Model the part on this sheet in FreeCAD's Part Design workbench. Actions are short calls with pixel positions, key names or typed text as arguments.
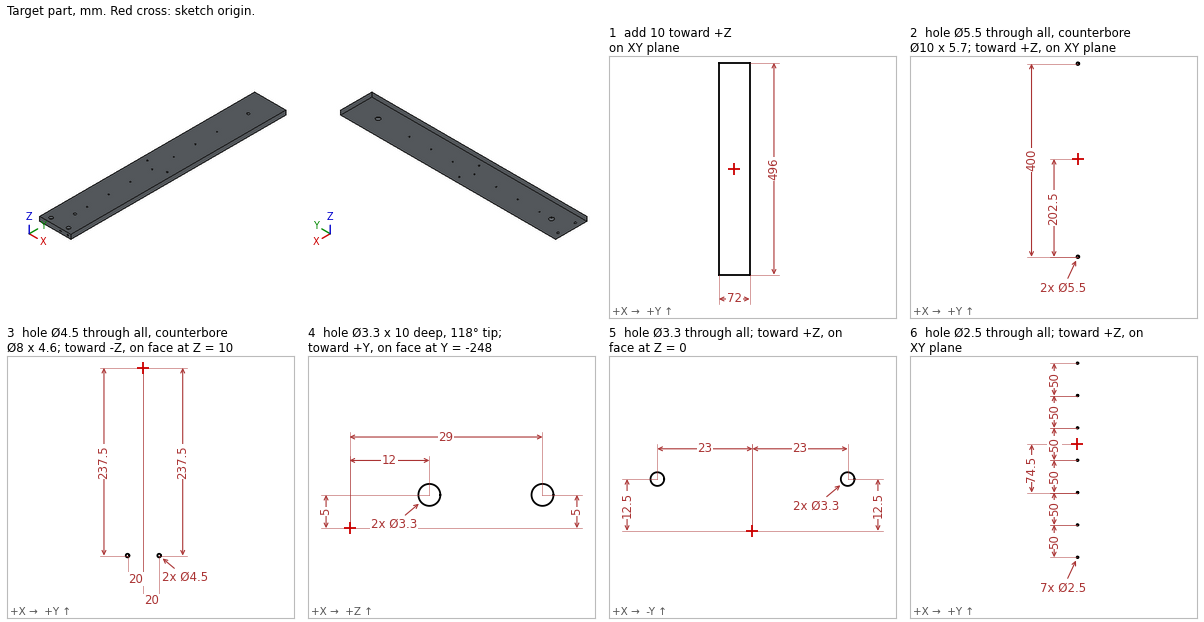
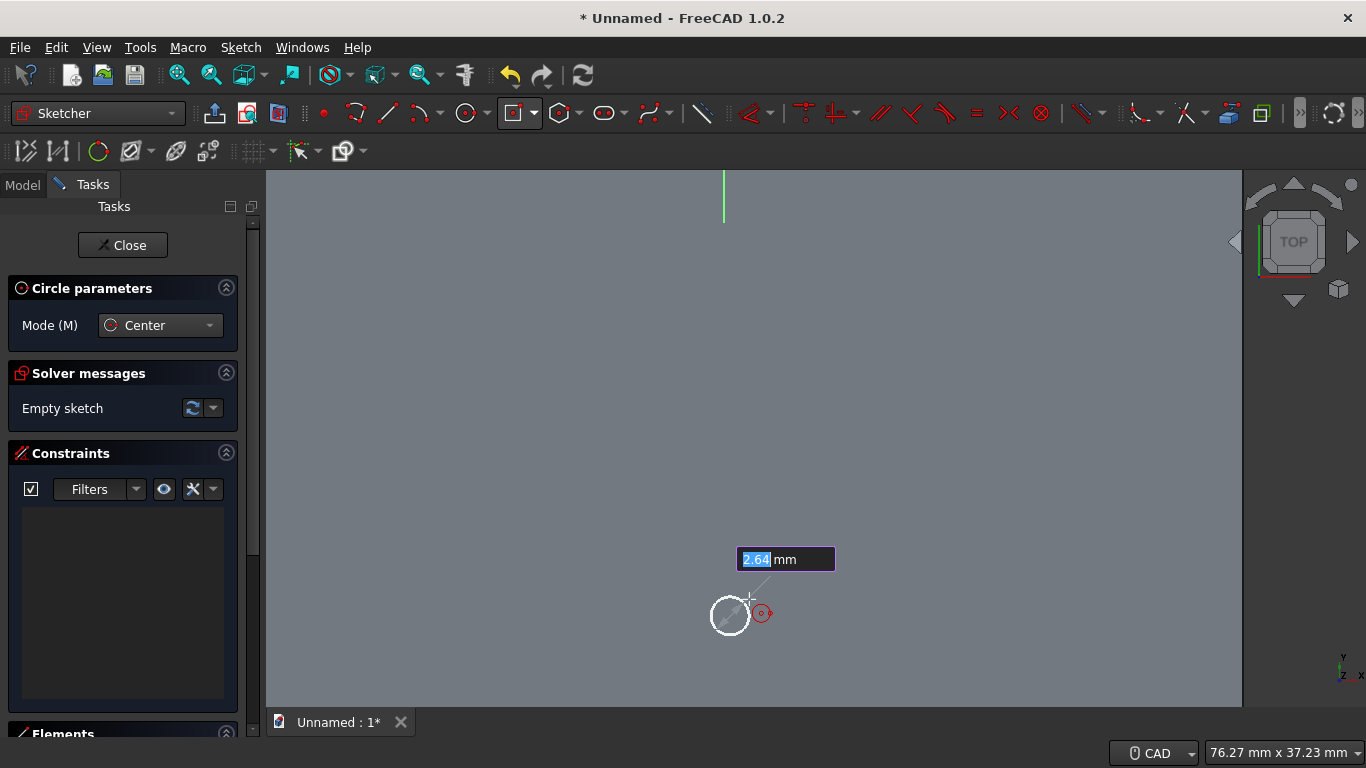
click(741, 593)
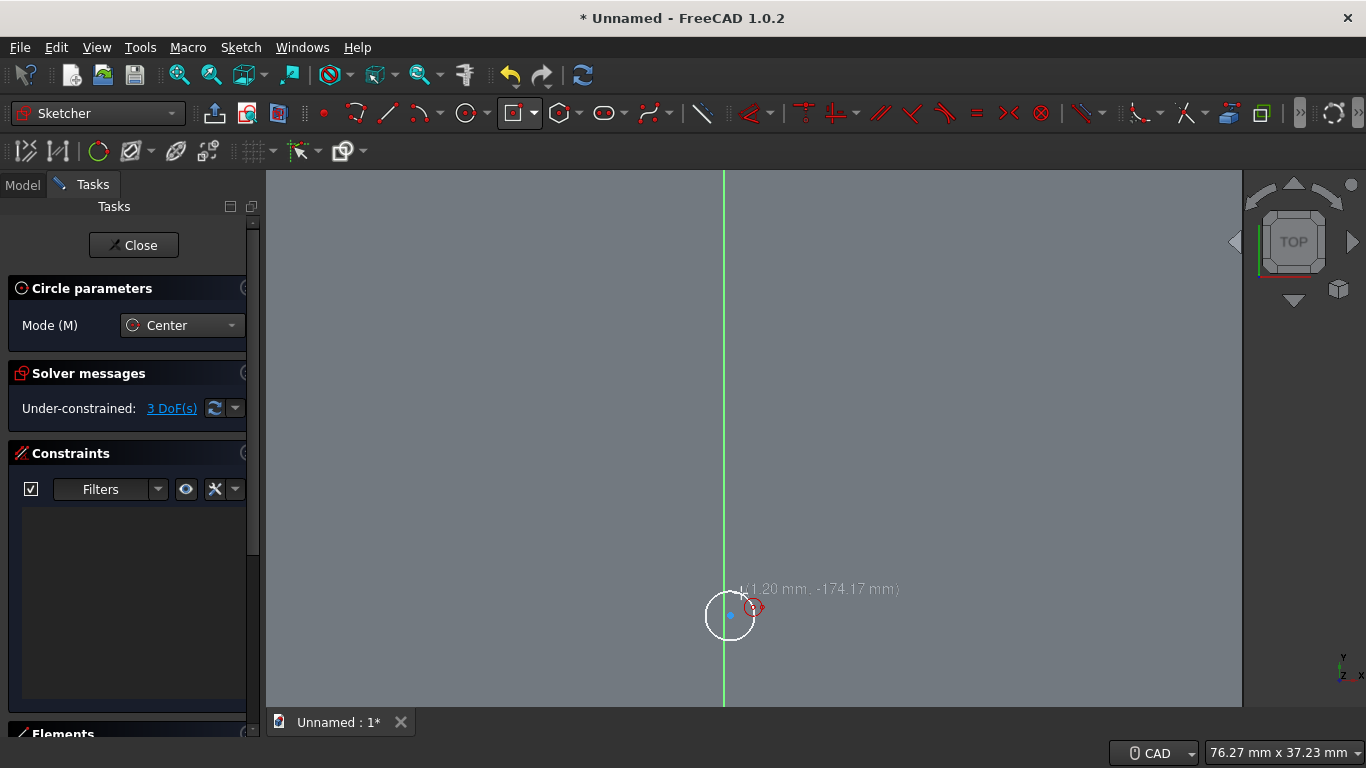
scroll(749, 599, down, 13)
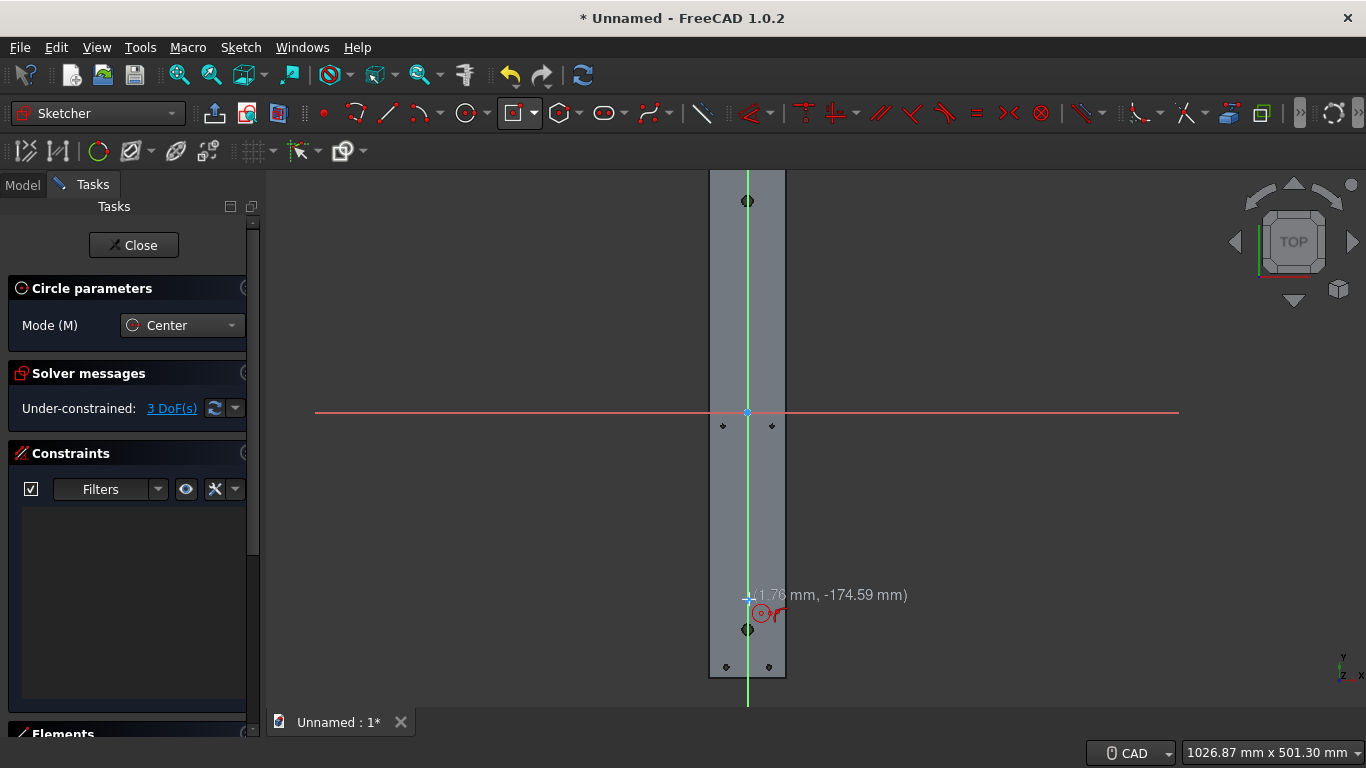
scroll(748, 546, up, 15)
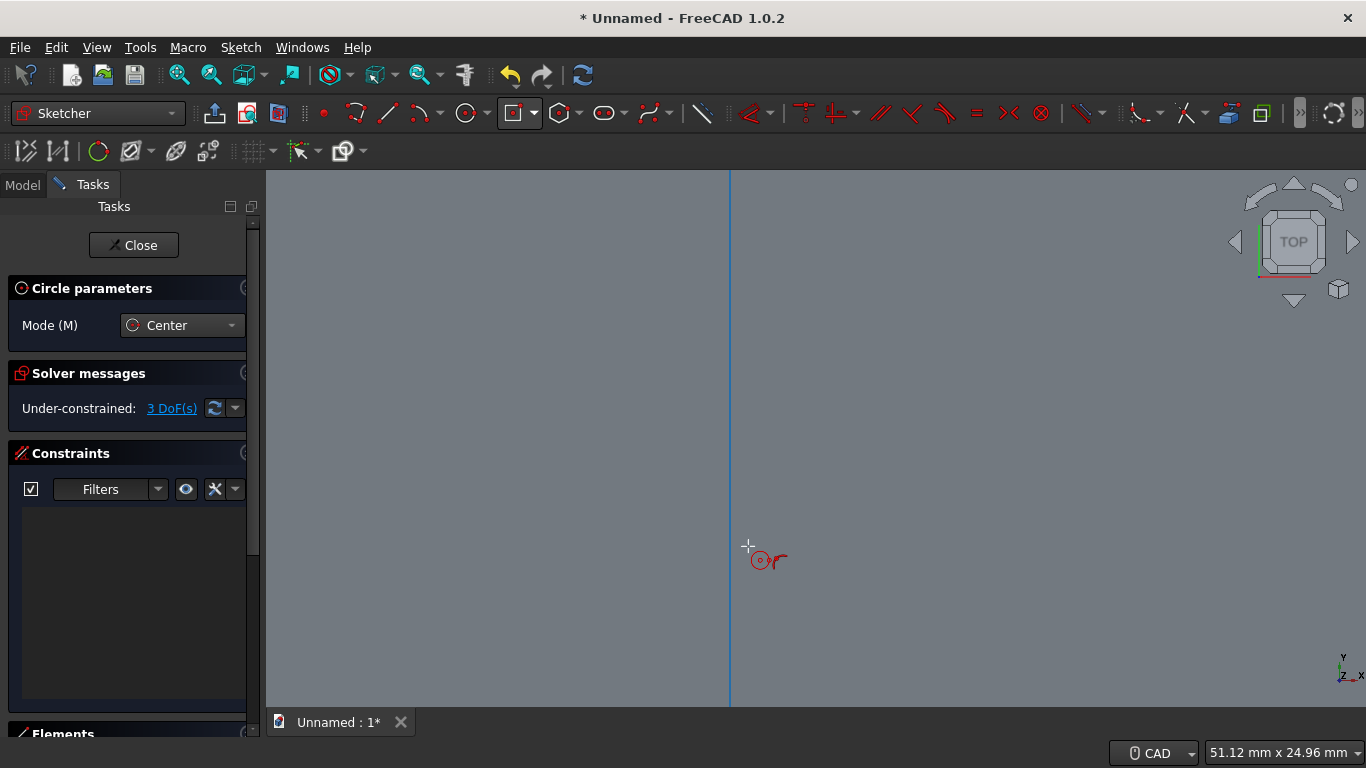
scroll(748, 546, down, 15)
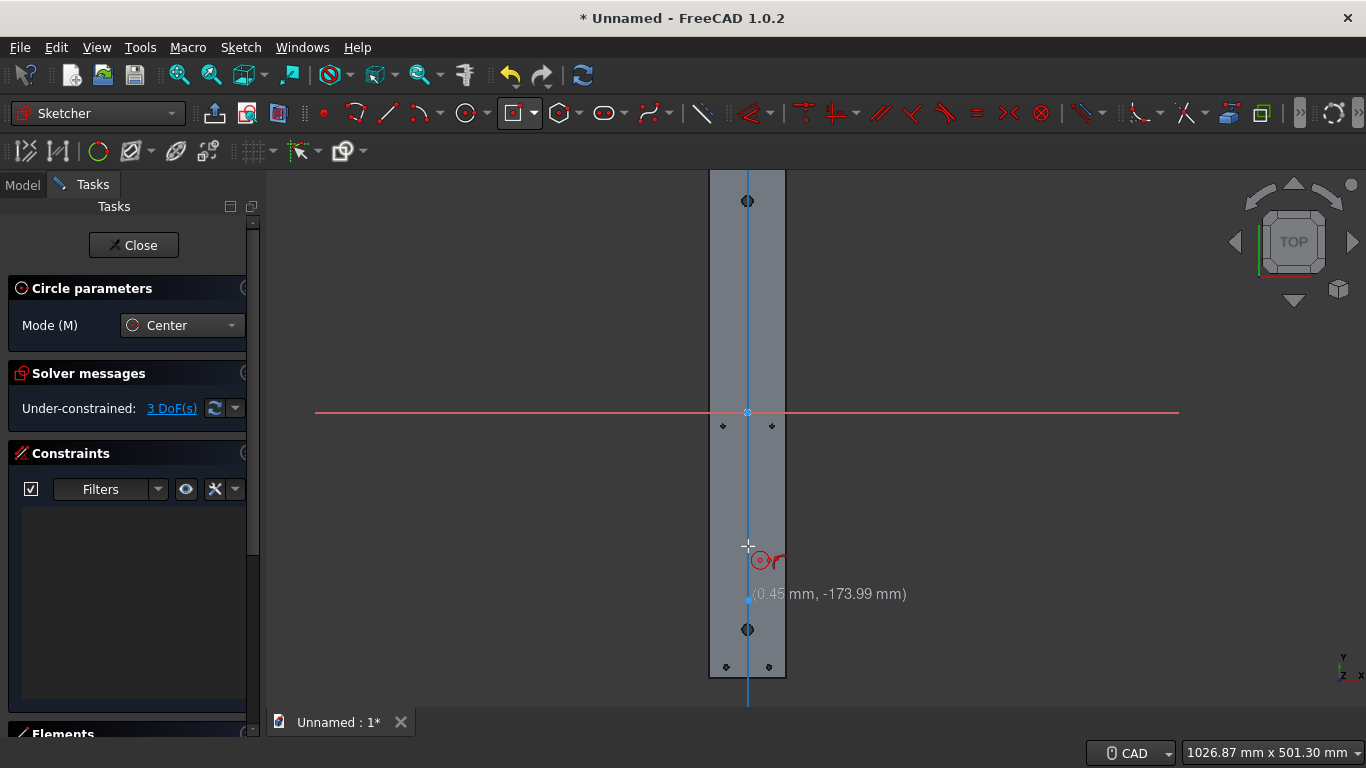
click(748, 546)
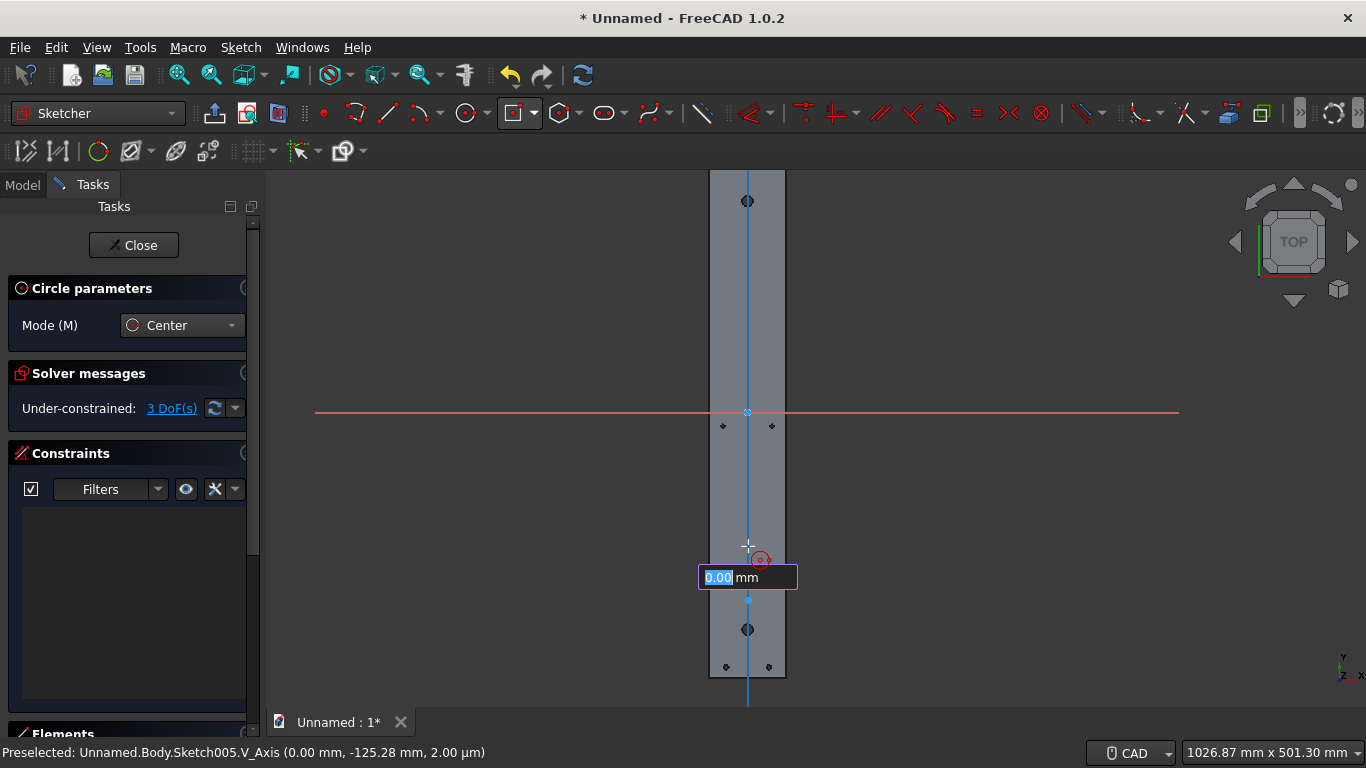
scroll(749, 546, up, 13)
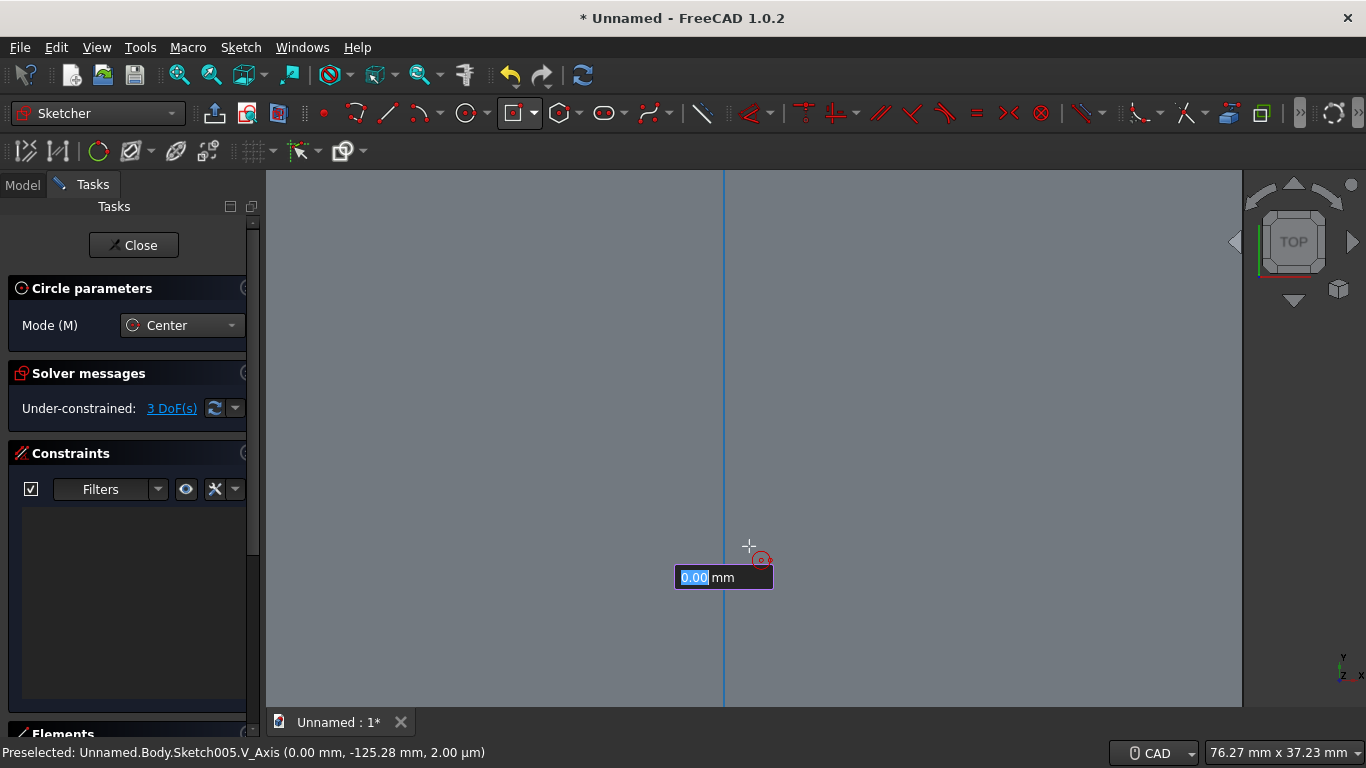
click(741, 533)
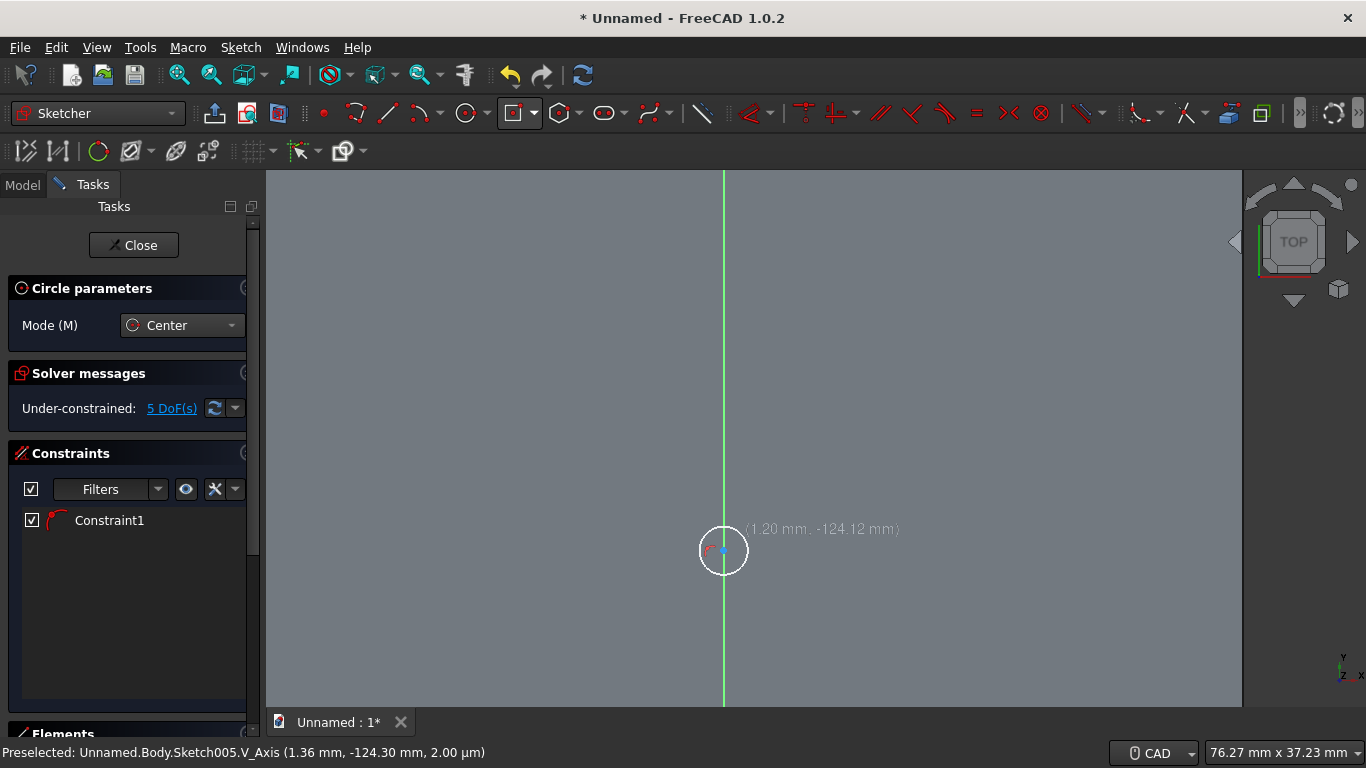
scroll(749, 546, down, 13)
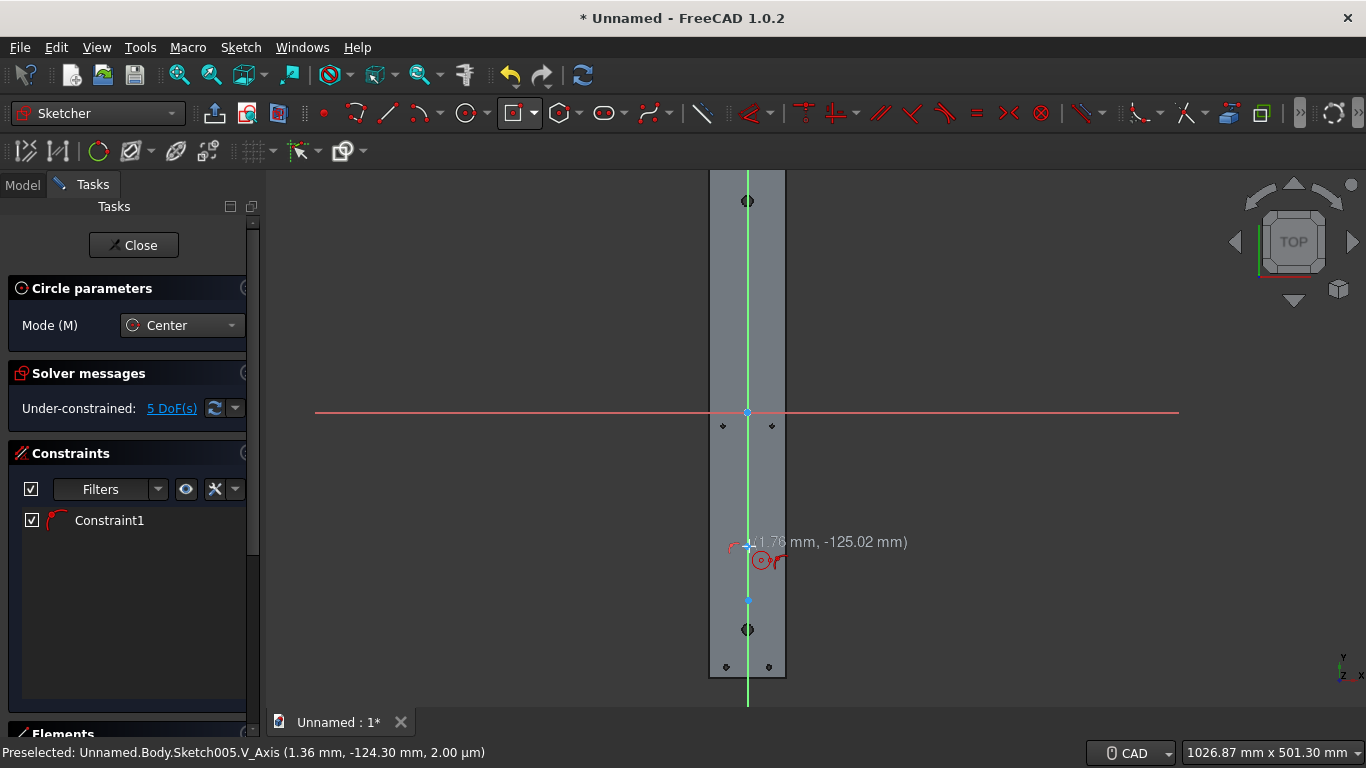
scroll(748, 493, up, 15)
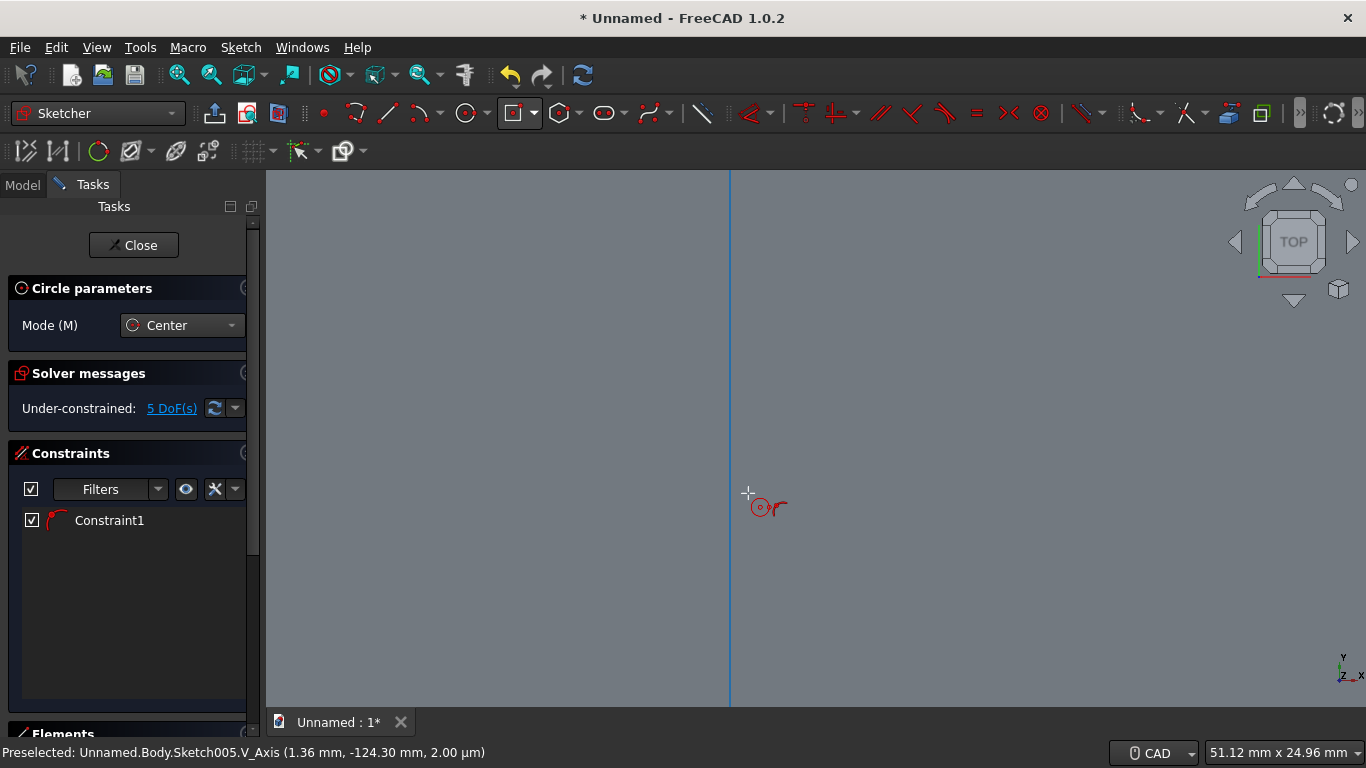
scroll(748, 493, down, 15)